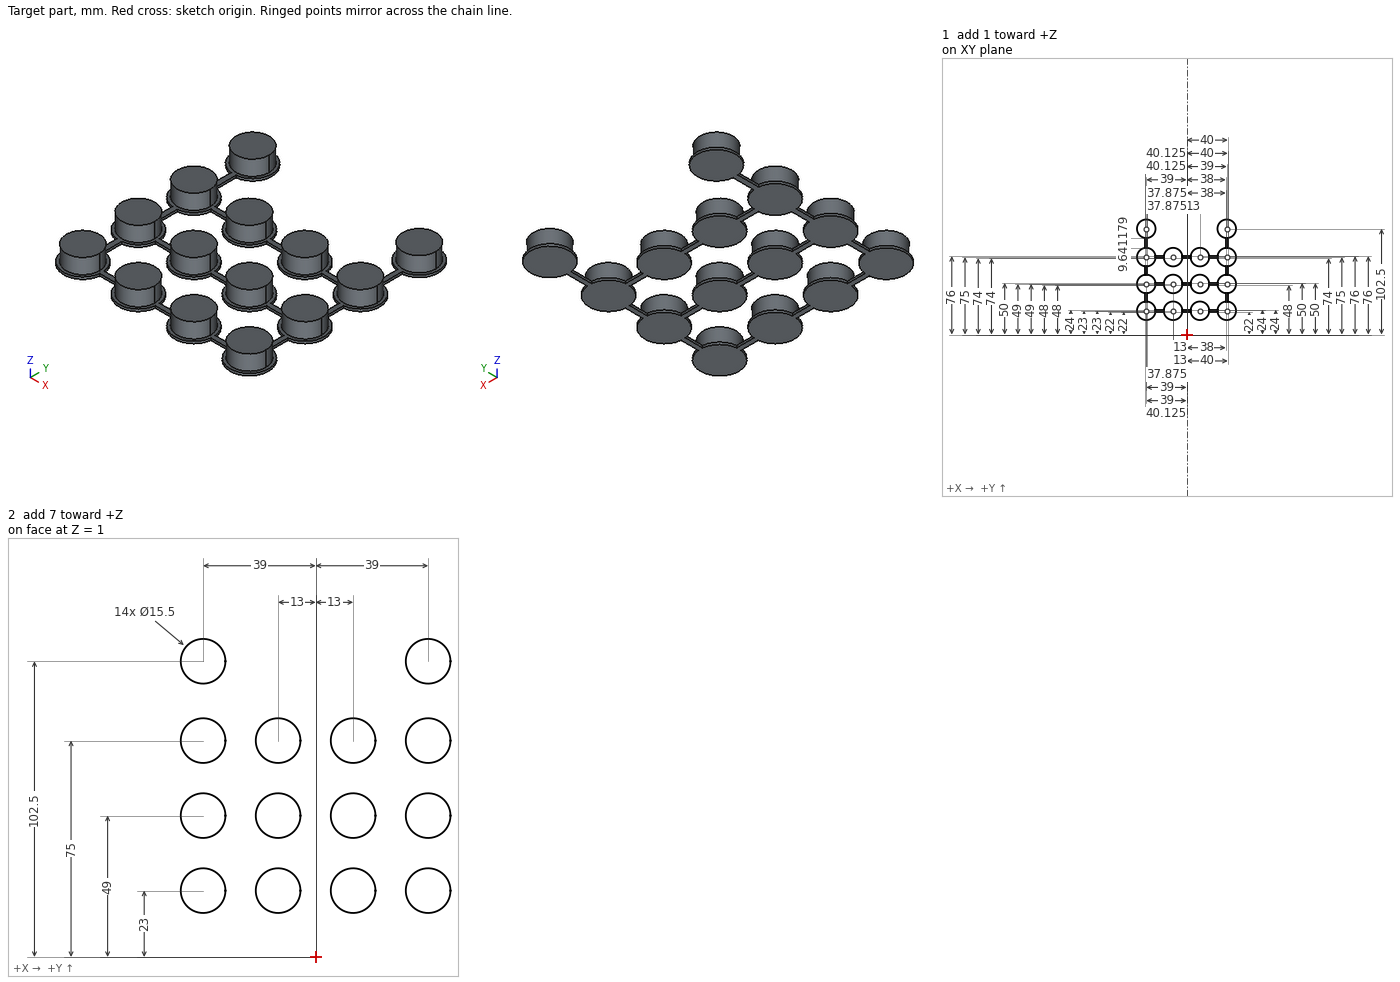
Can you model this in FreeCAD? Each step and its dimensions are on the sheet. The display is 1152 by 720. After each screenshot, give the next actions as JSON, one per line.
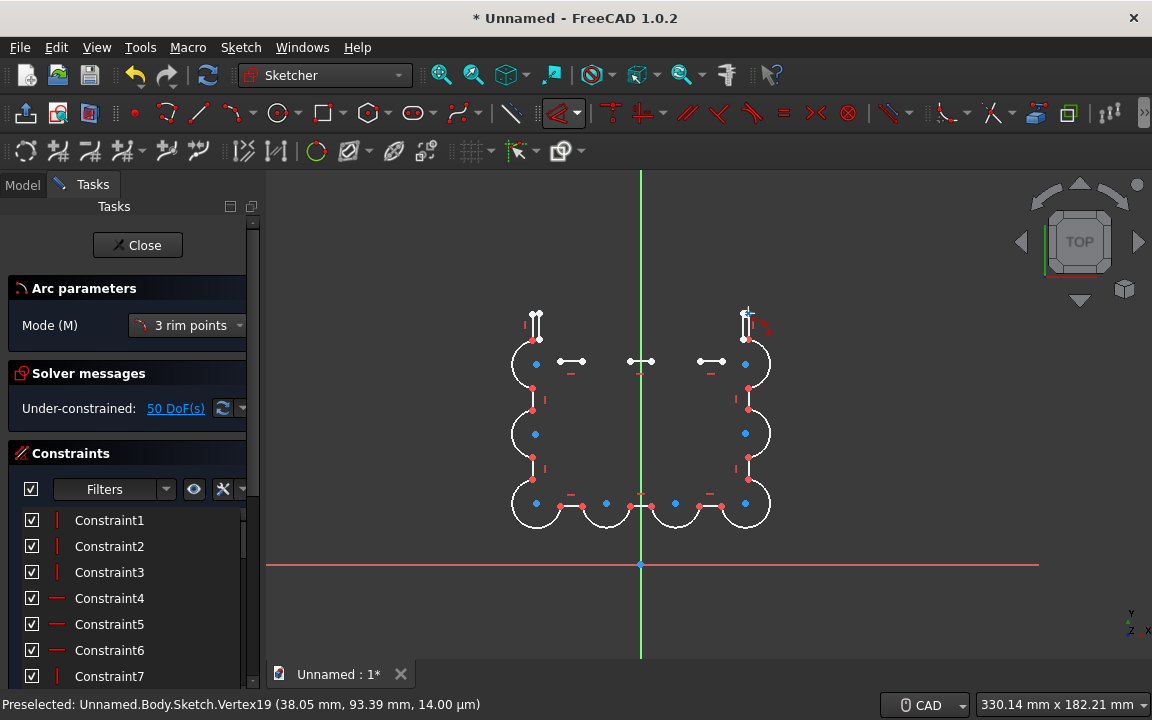
{"action": "left_click", "coordinate": [746, 265]}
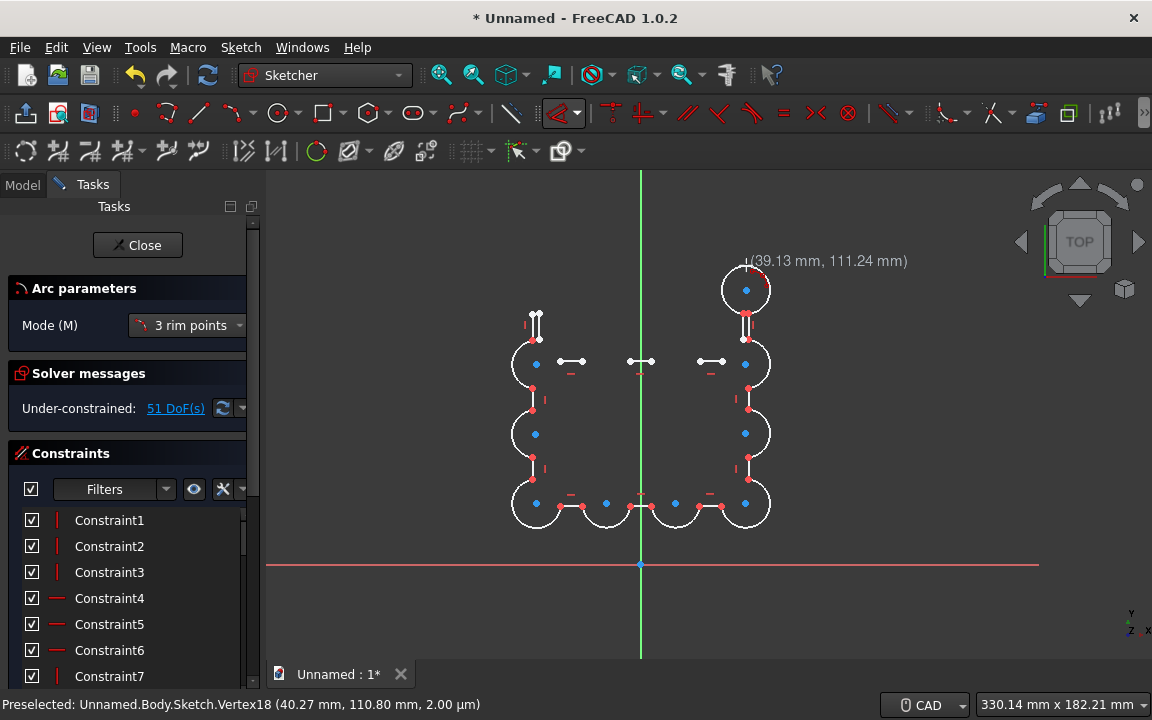
{"action": "scroll", "coordinate": [743, 339], "scroll_direction": "up", "scroll_amount": 6}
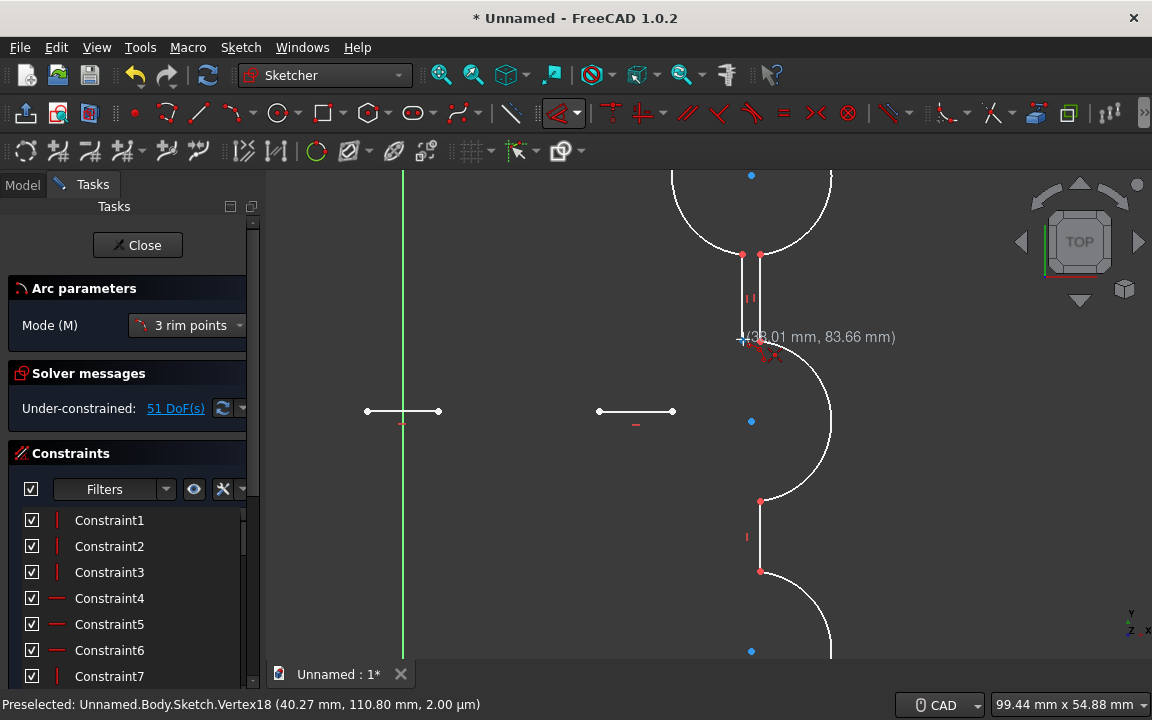
{"action": "left_click", "coordinate": [742, 340]}
{"action": "left_click", "coordinate": [672, 412]}
{"action": "left_click", "coordinate": [694, 362]}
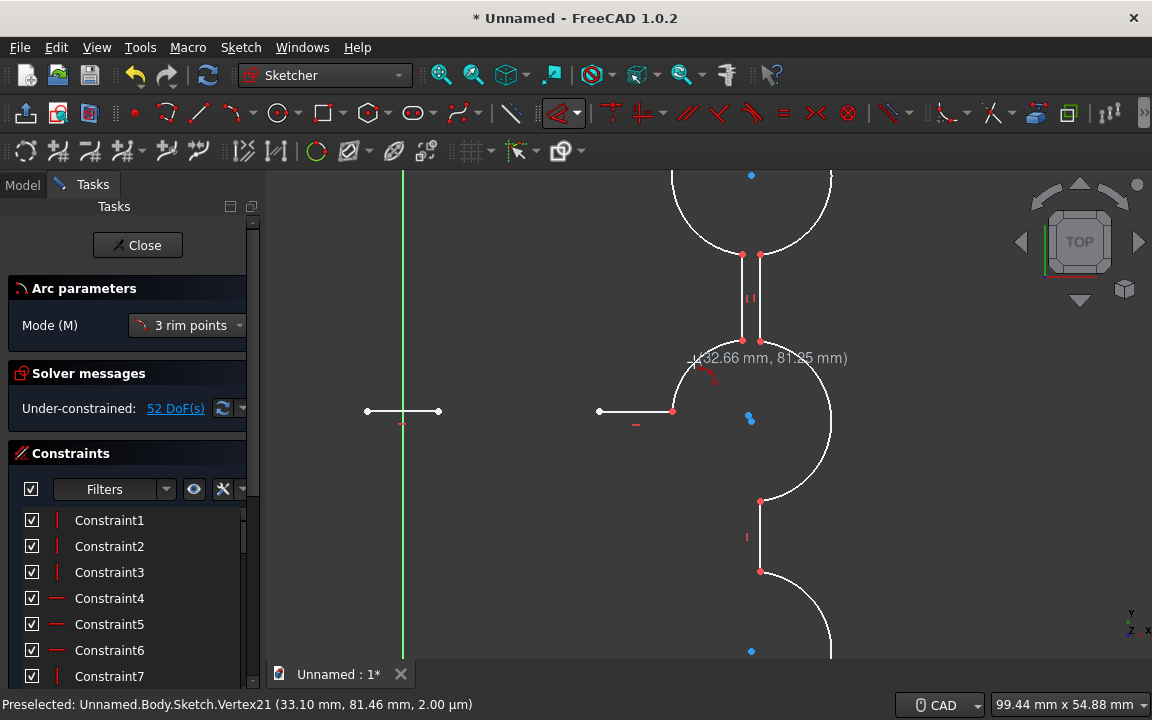
{"action": "left_click", "coordinate": [600, 412]}
{"action": "left_click", "coordinate": [438, 411]}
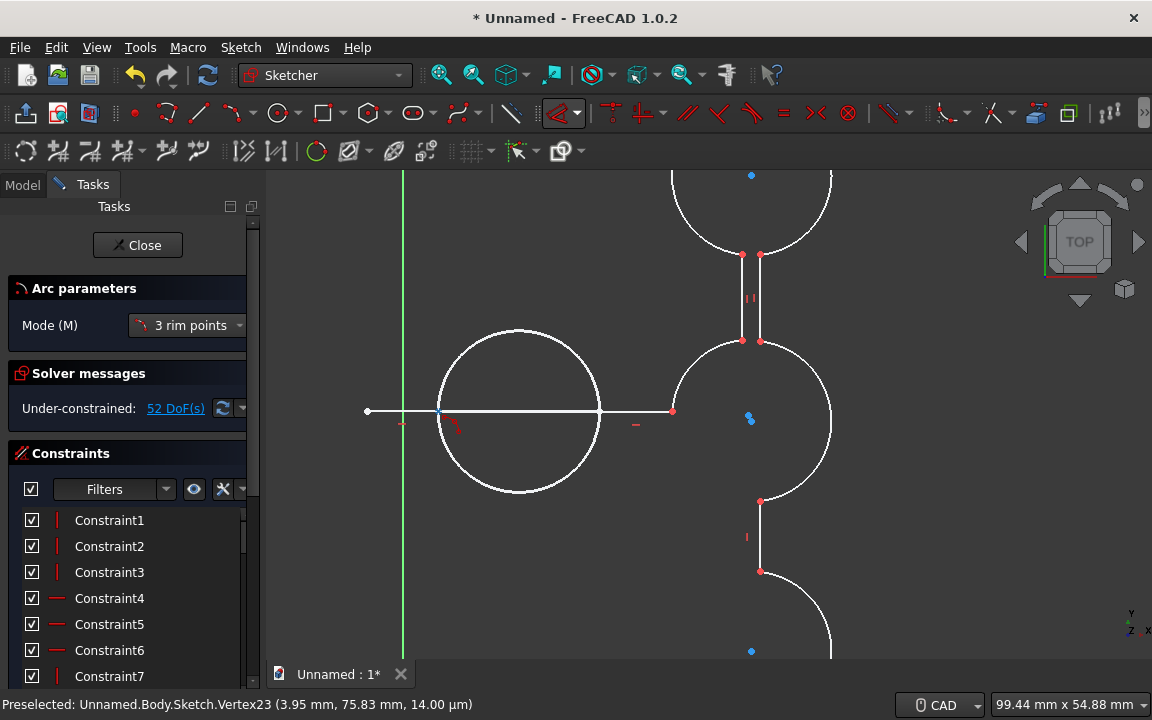
{"action": "scroll", "coordinate": [743, 339], "scroll_direction": "down", "scroll_amount": 6}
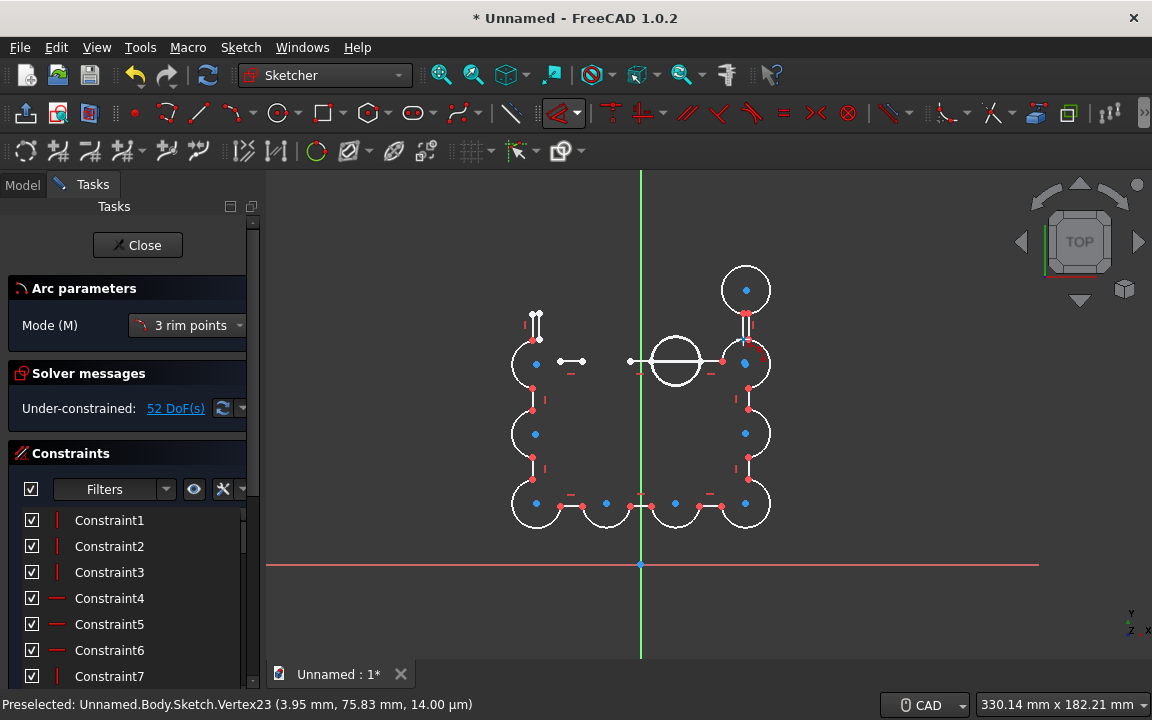
{"action": "left_click", "coordinate": [676, 339]}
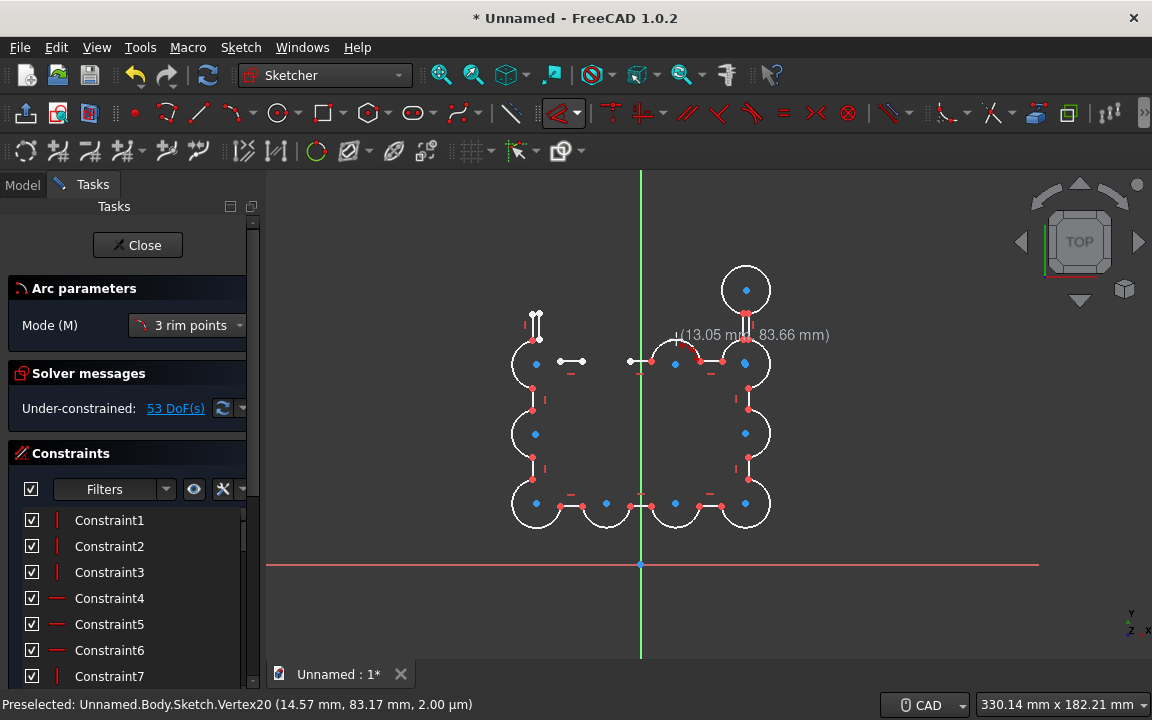
{"action": "scroll", "coordinate": [630, 361], "scroll_direction": "up", "scroll_amount": 2}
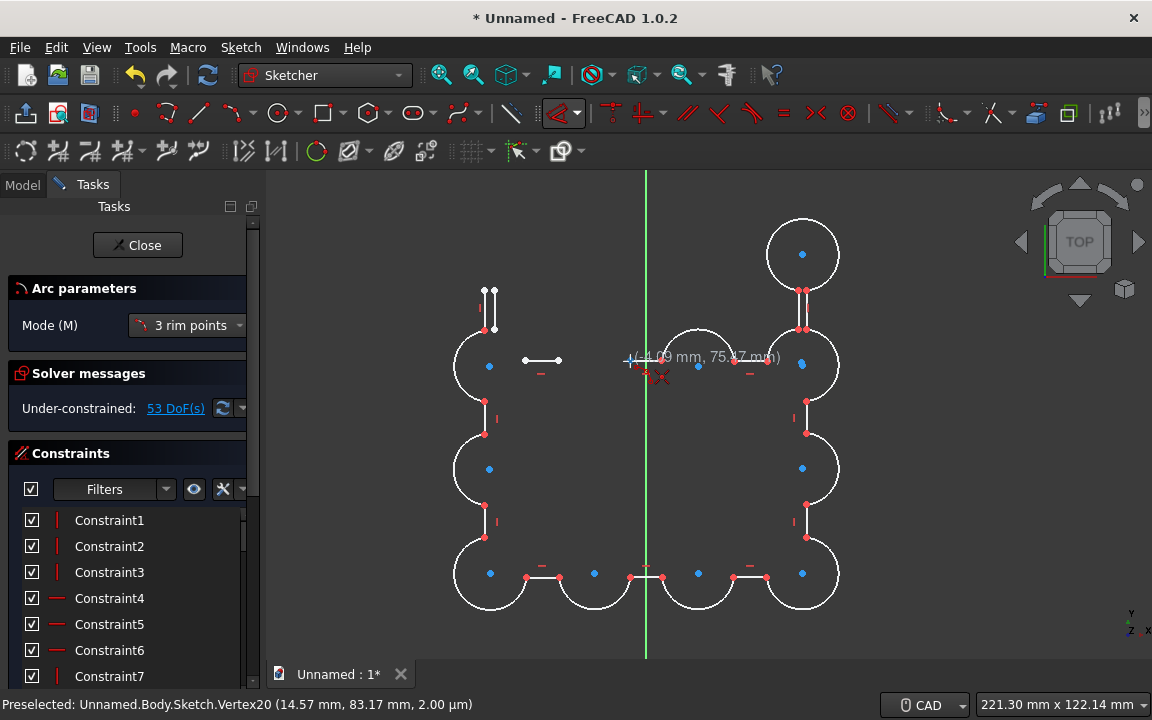
{"action": "left_click", "coordinate": [630, 361]}
{"action": "left_click", "coordinate": [558, 361]}
{"action": "left_click", "coordinate": [594, 328]}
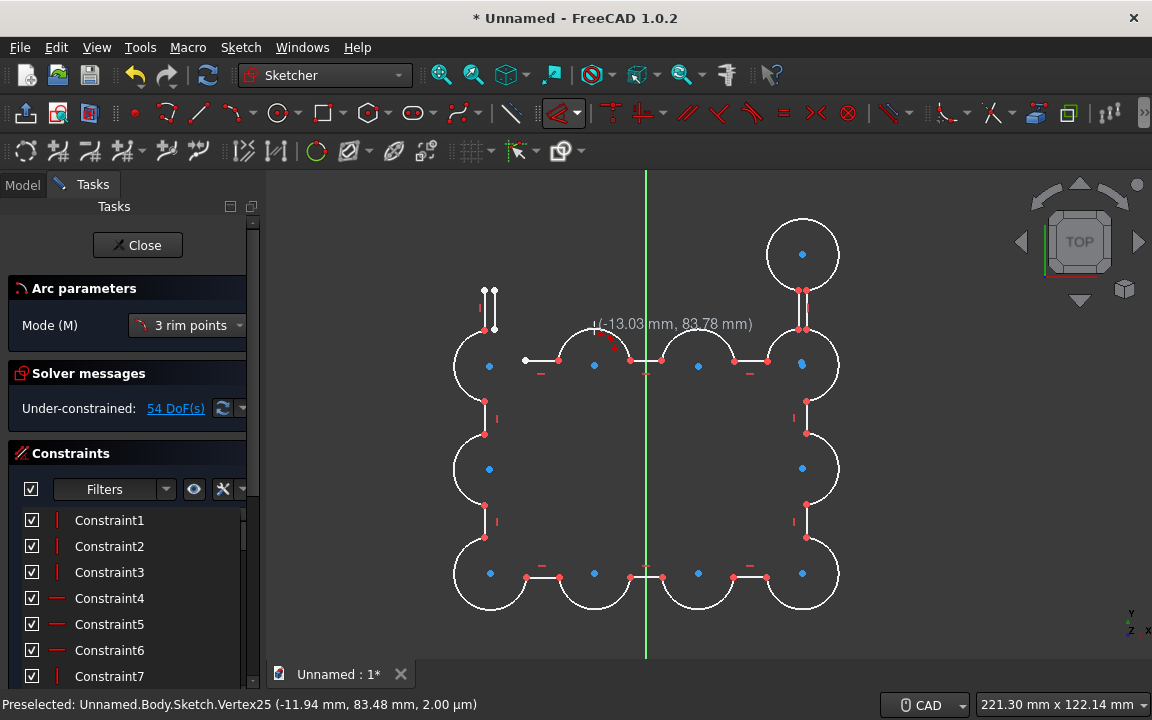
{"action": "left_click", "coordinate": [526, 361]}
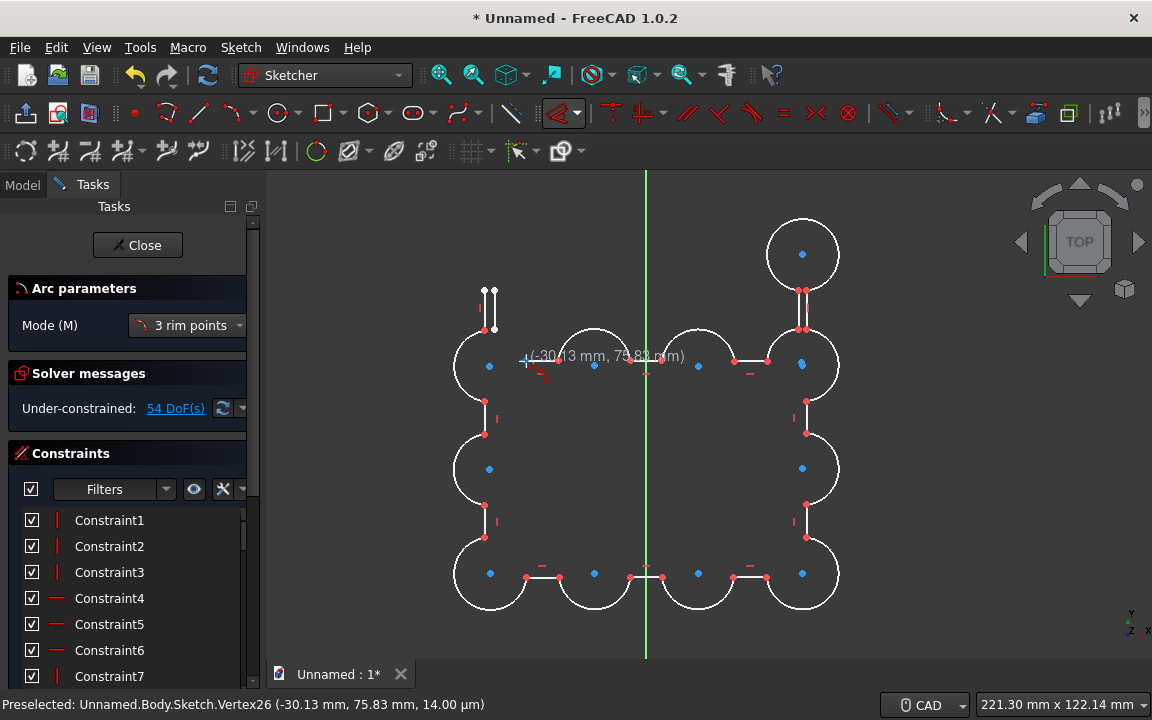
{"action": "scroll", "coordinate": [495, 328], "scroll_direction": "up", "scroll_amount": 3}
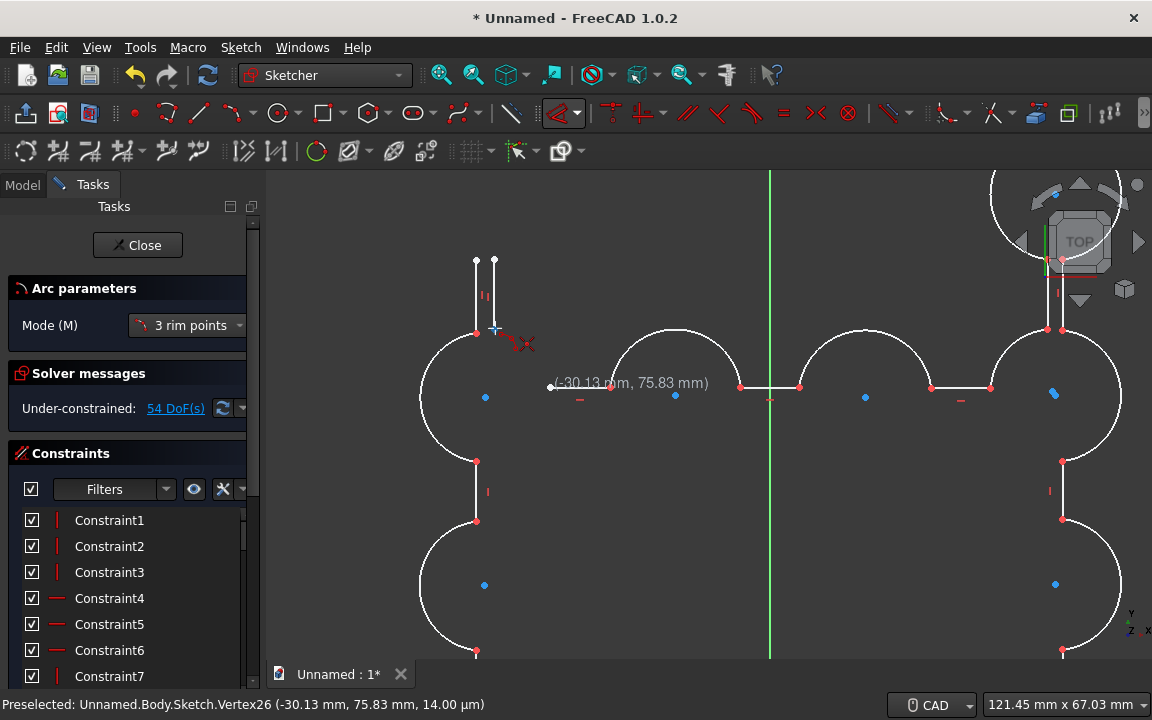
{"action": "left_click", "coordinate": [494, 330]}
{"action": "left_click", "coordinate": [533, 348]}